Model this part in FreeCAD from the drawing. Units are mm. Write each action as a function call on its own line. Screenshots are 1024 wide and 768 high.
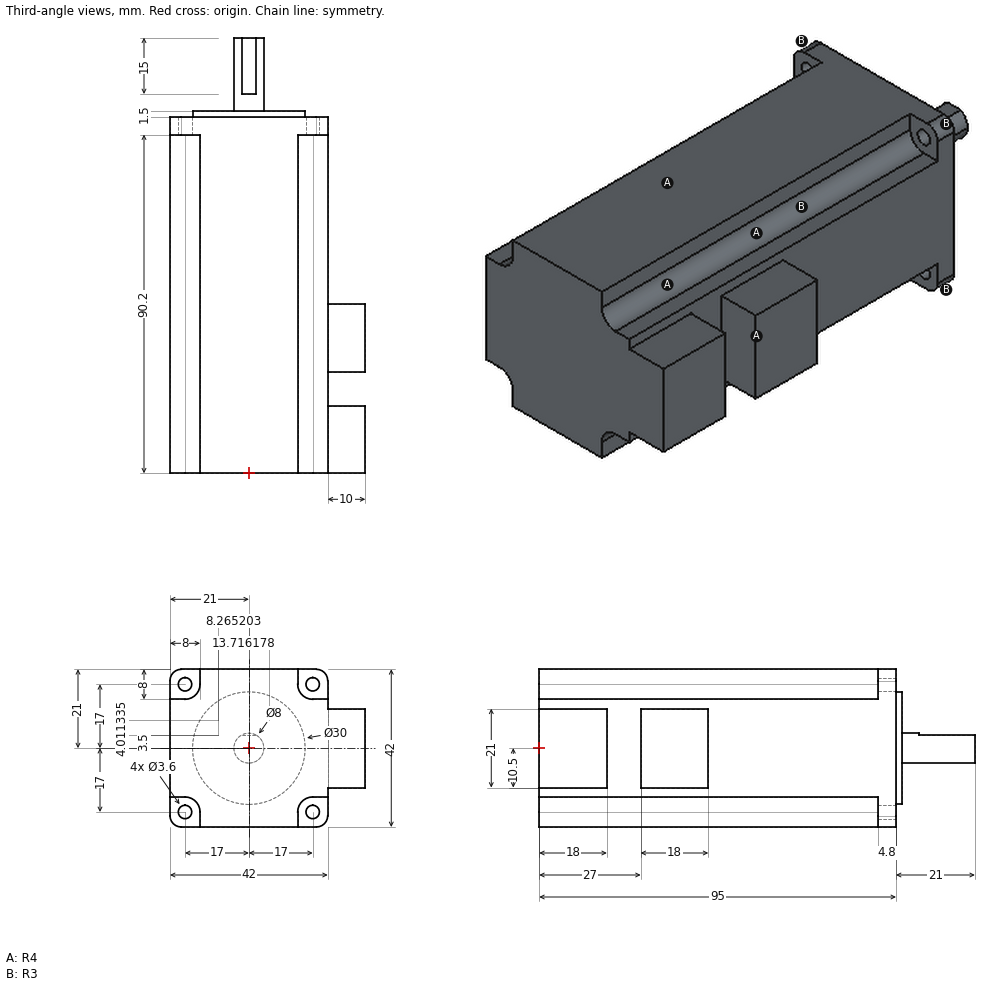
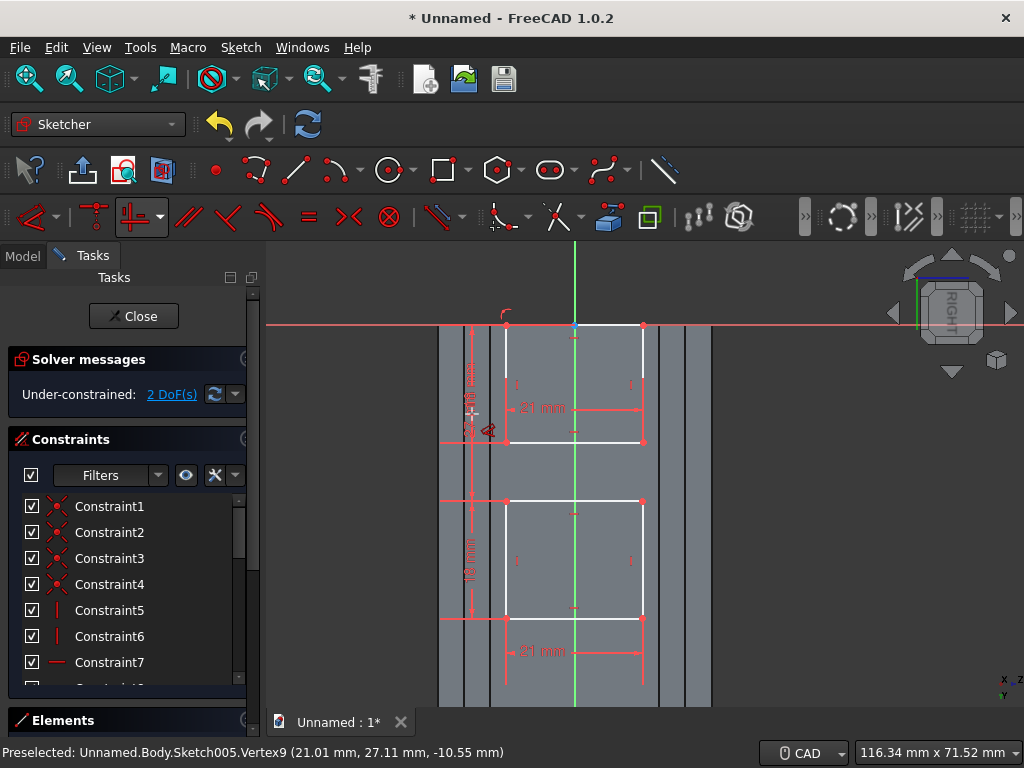
click(506, 325)
click(540, 291)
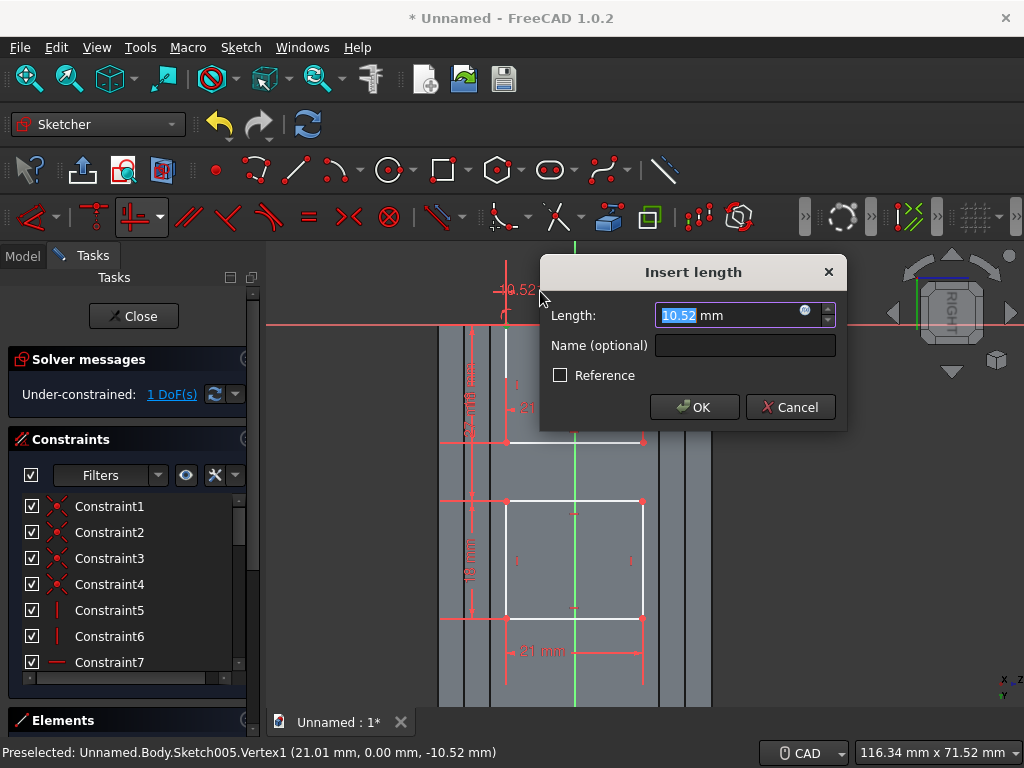
text(10.5)
key(Return)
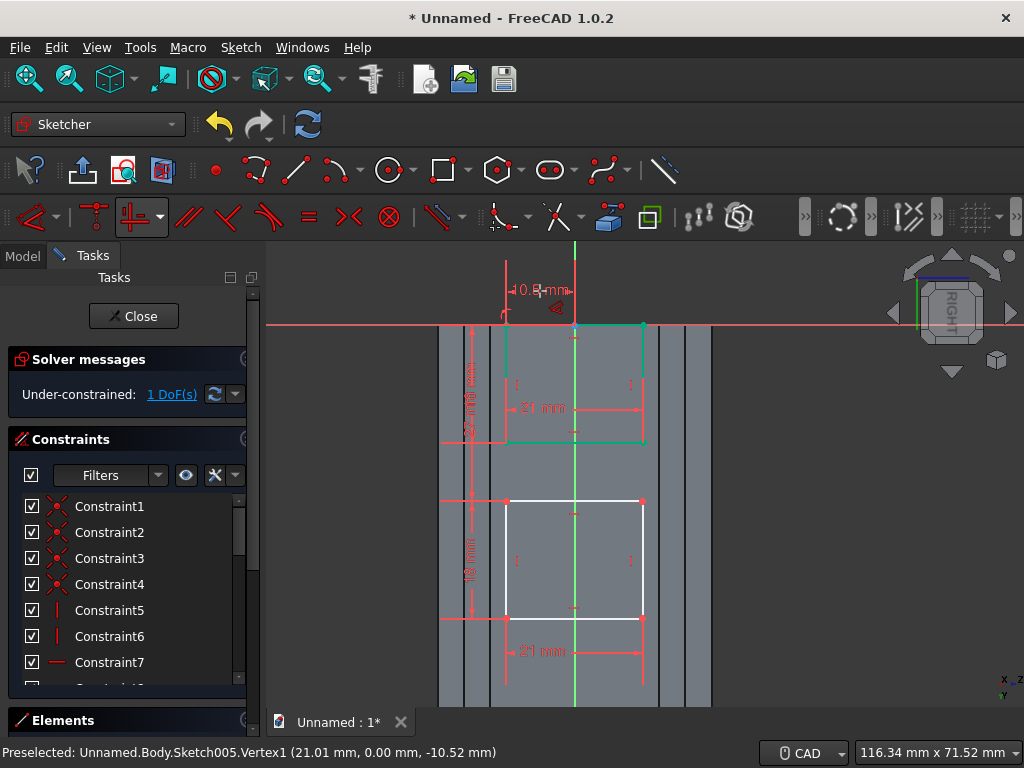
click(506, 501)
click(540, 535)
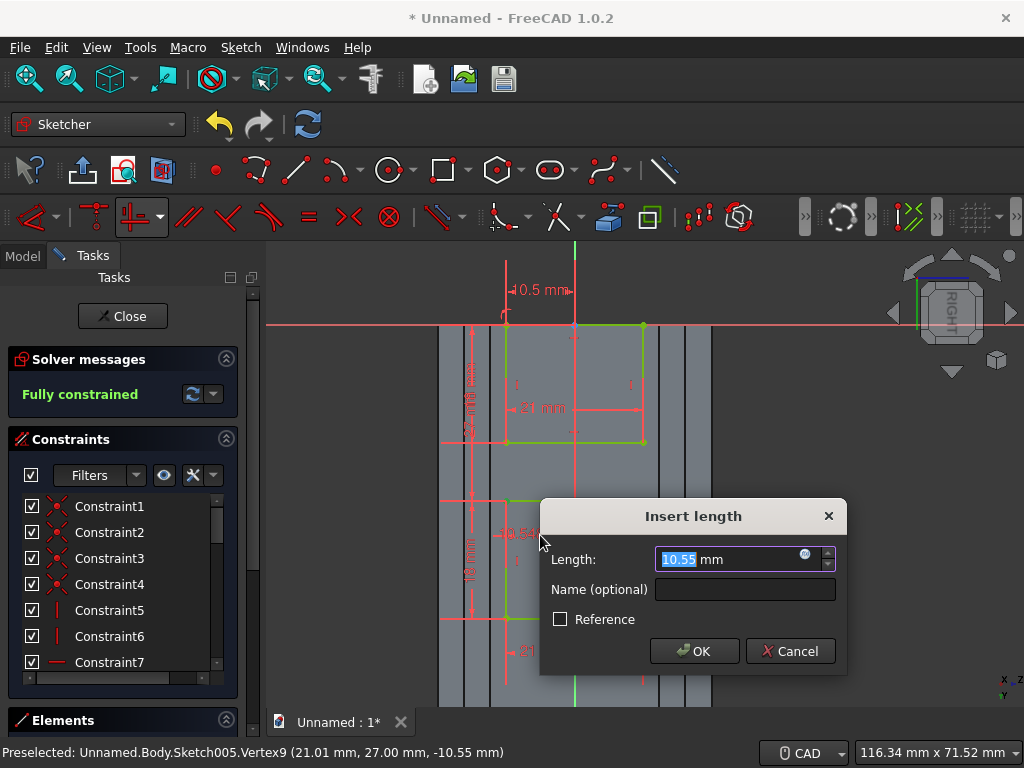
text(10.5)
key(Return)
key(Escape)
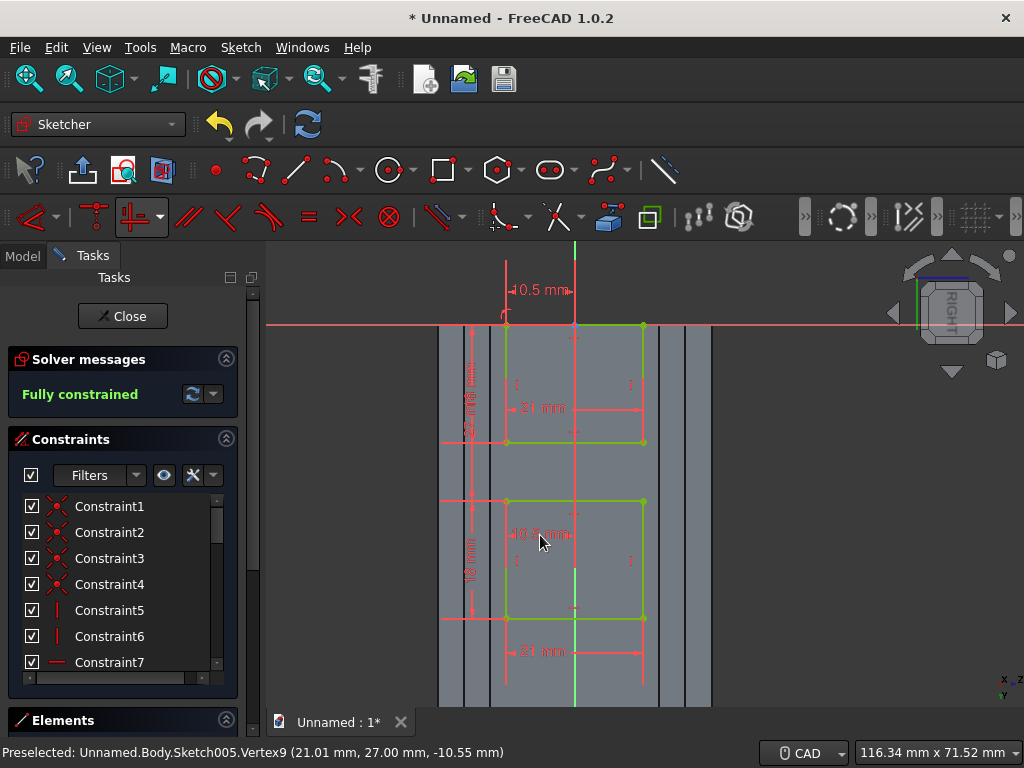
click(123, 316)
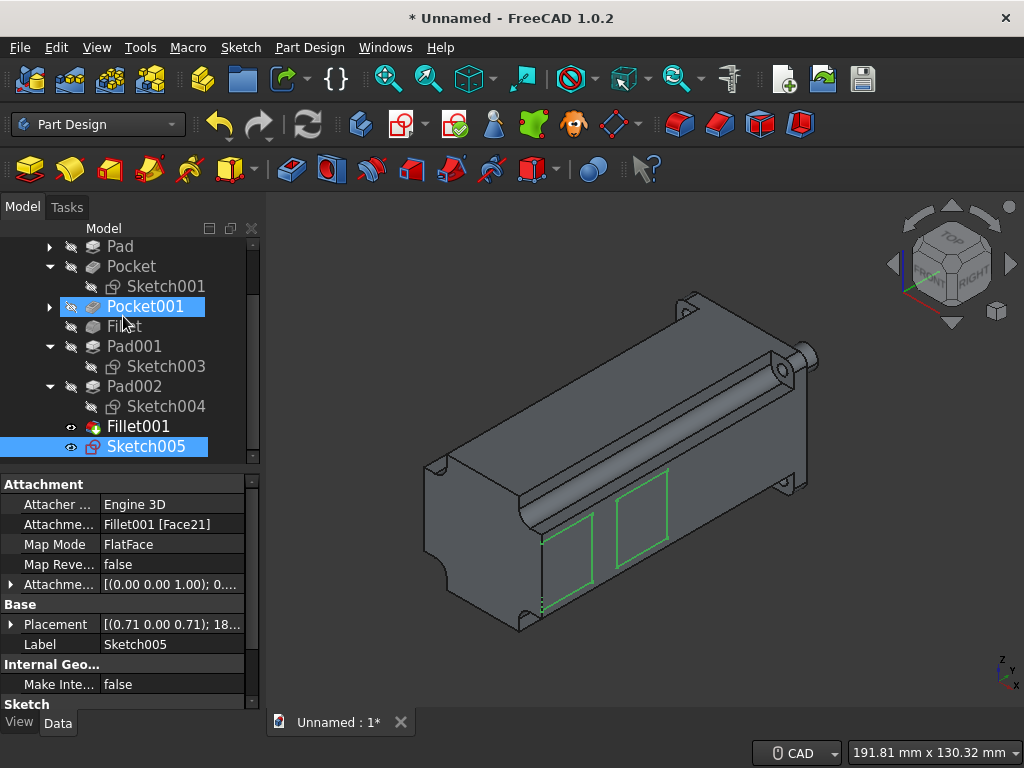
click(30, 170)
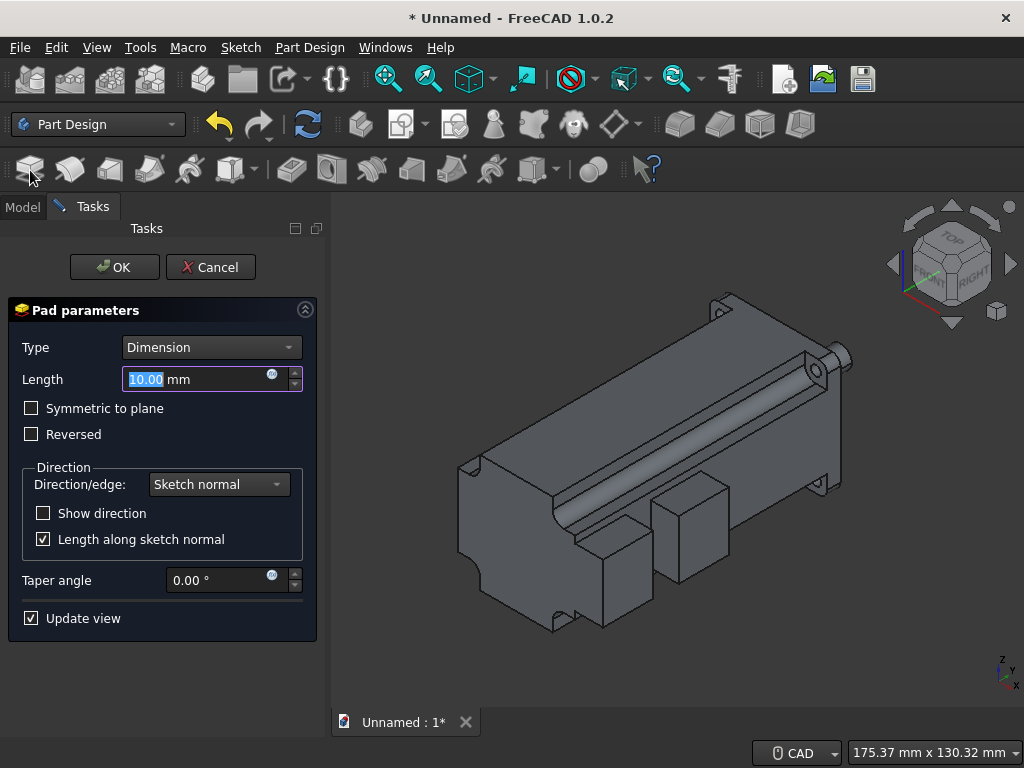
text(10)
key(Tab)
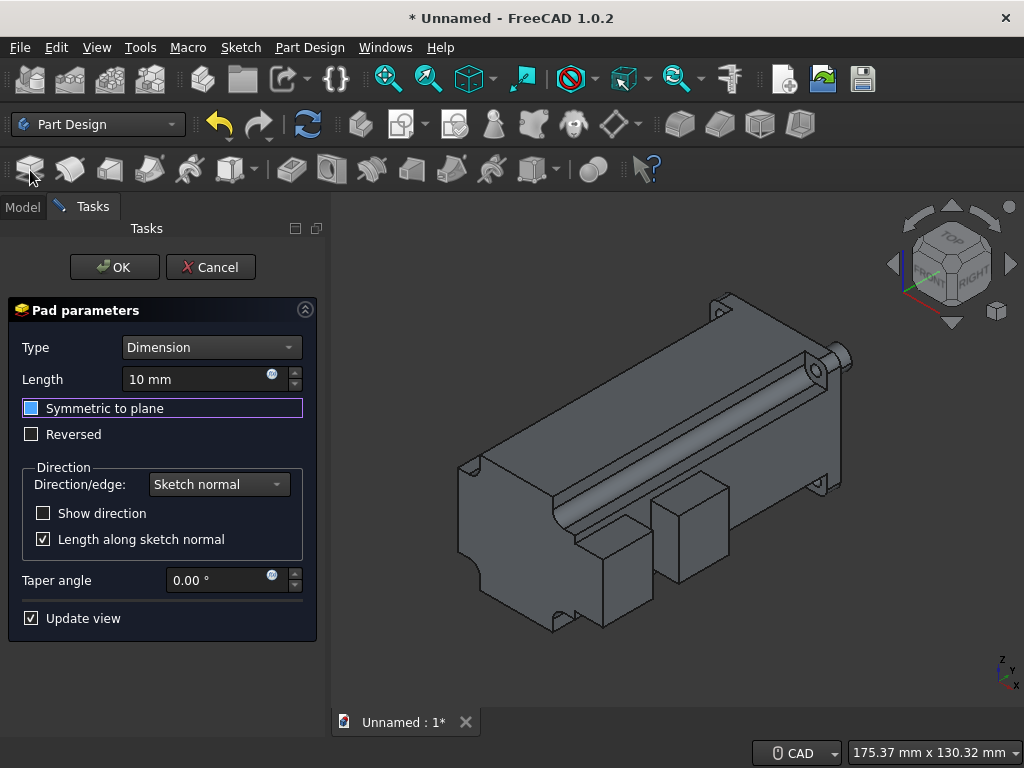
click(115, 267)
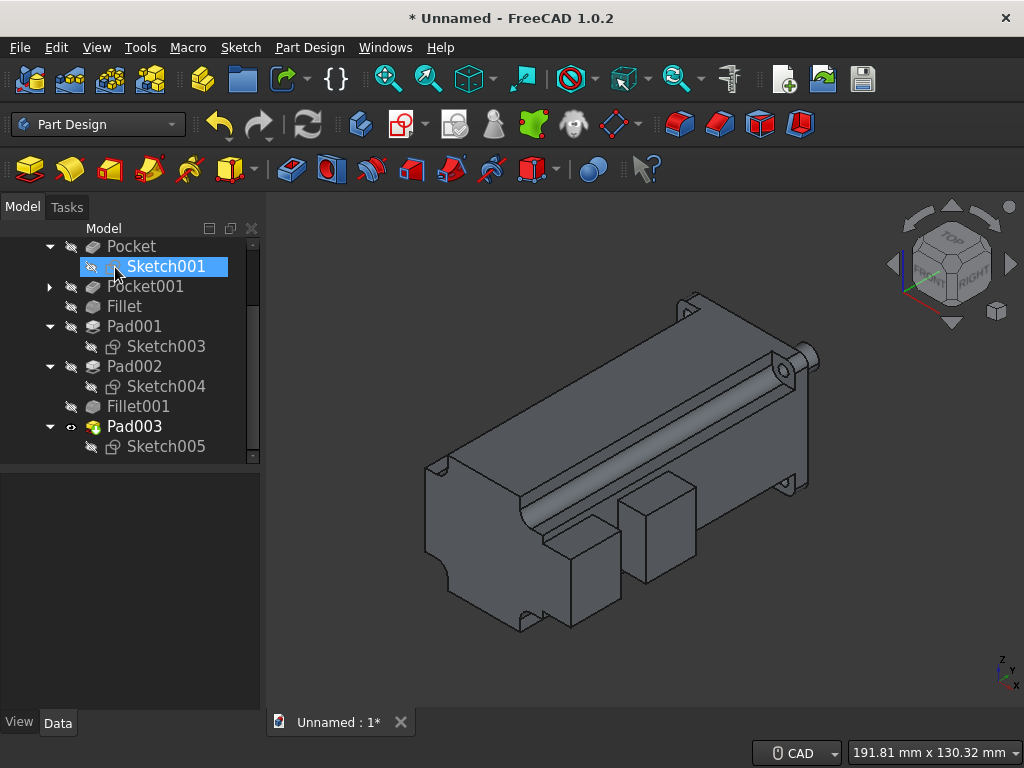
key(4)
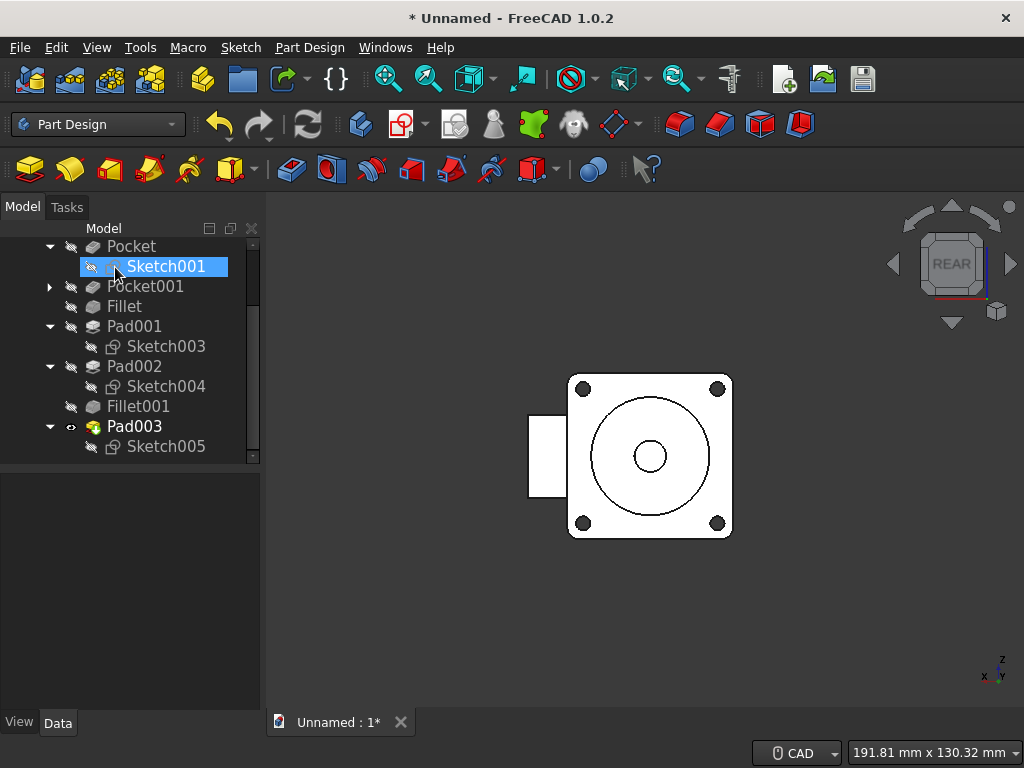
key(v)
key(f)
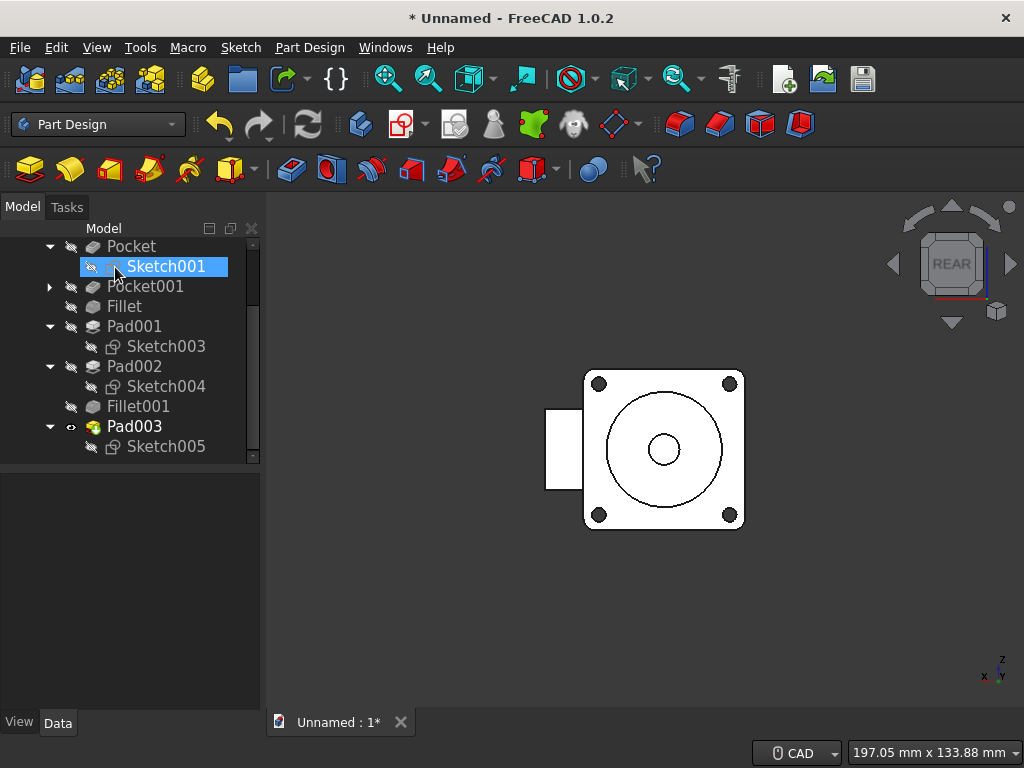
click(664, 449)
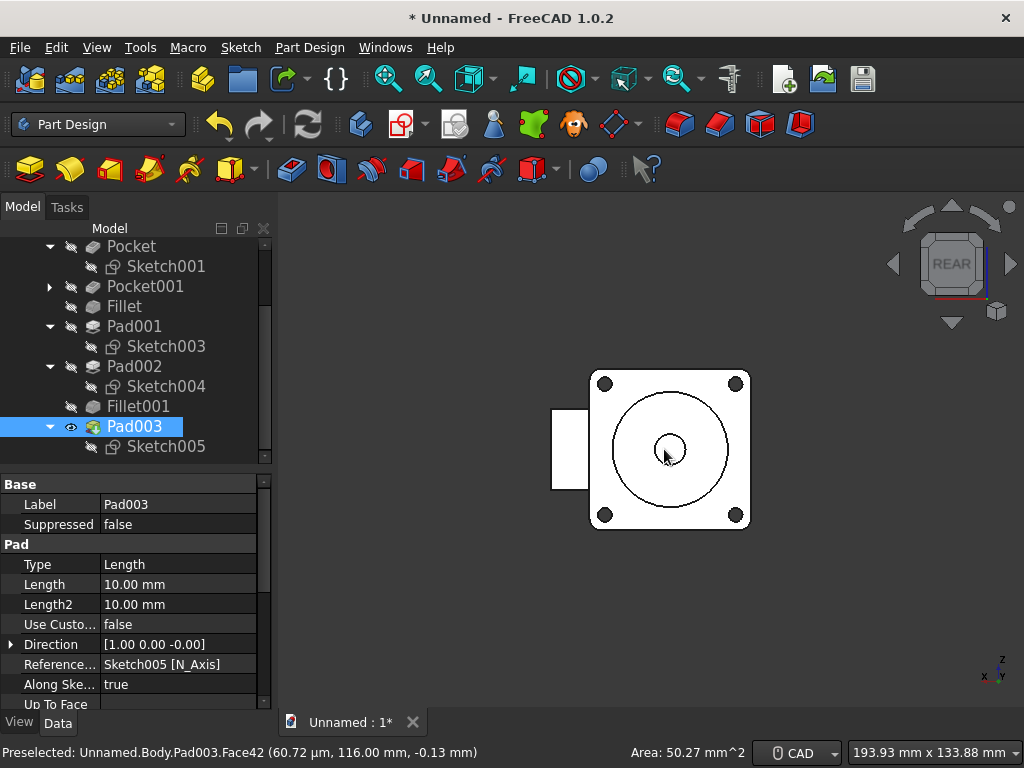
click(402, 124)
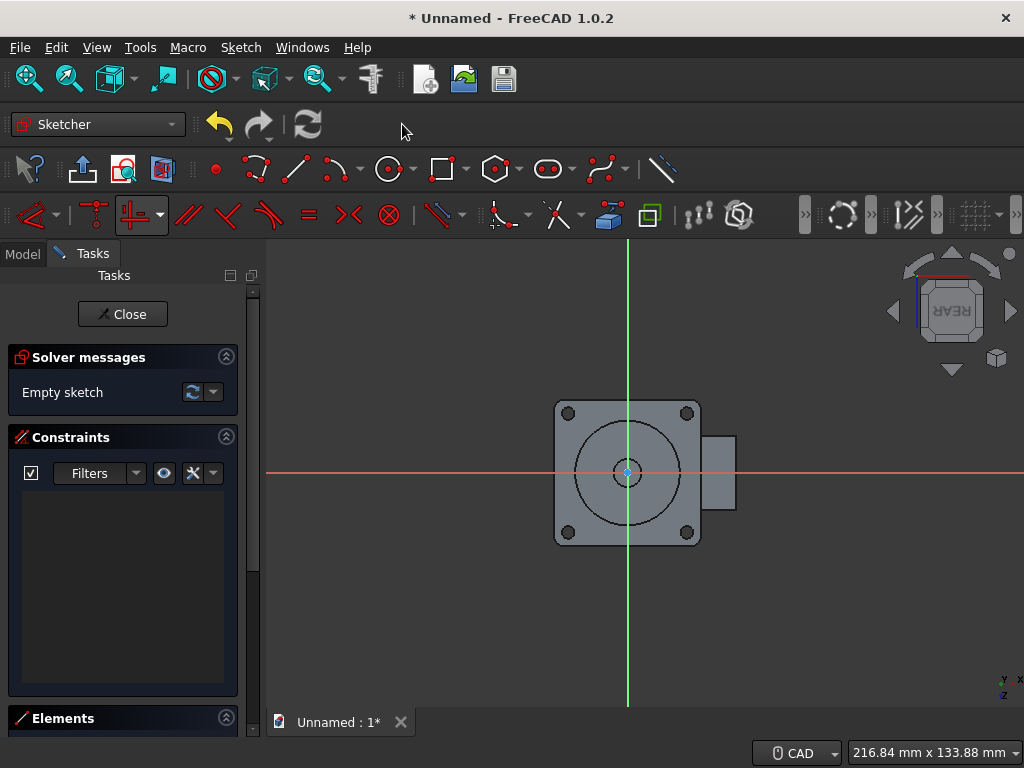
scroll(628, 488, up, 11)